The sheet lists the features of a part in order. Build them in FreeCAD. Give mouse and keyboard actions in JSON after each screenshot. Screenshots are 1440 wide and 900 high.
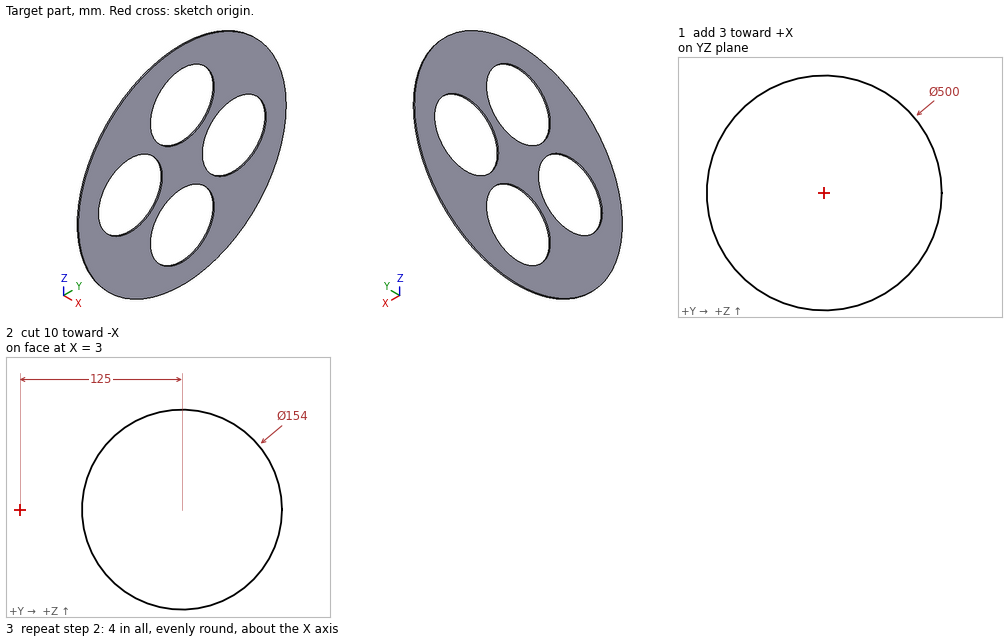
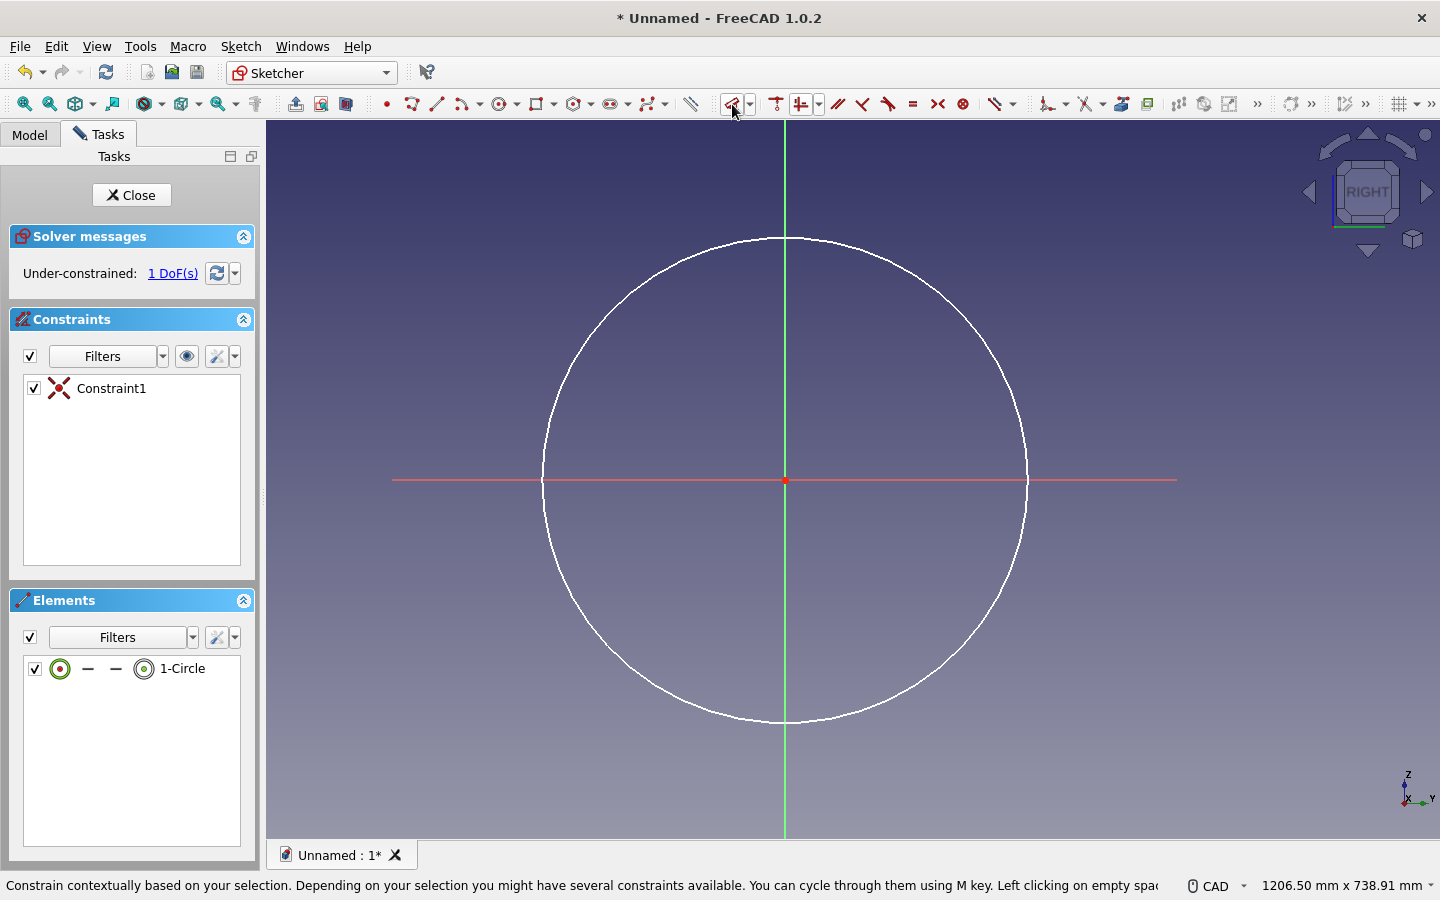
{"action": "left_click", "coordinate": [956, 308]}
{"action": "left_click", "coordinate": [979, 285]}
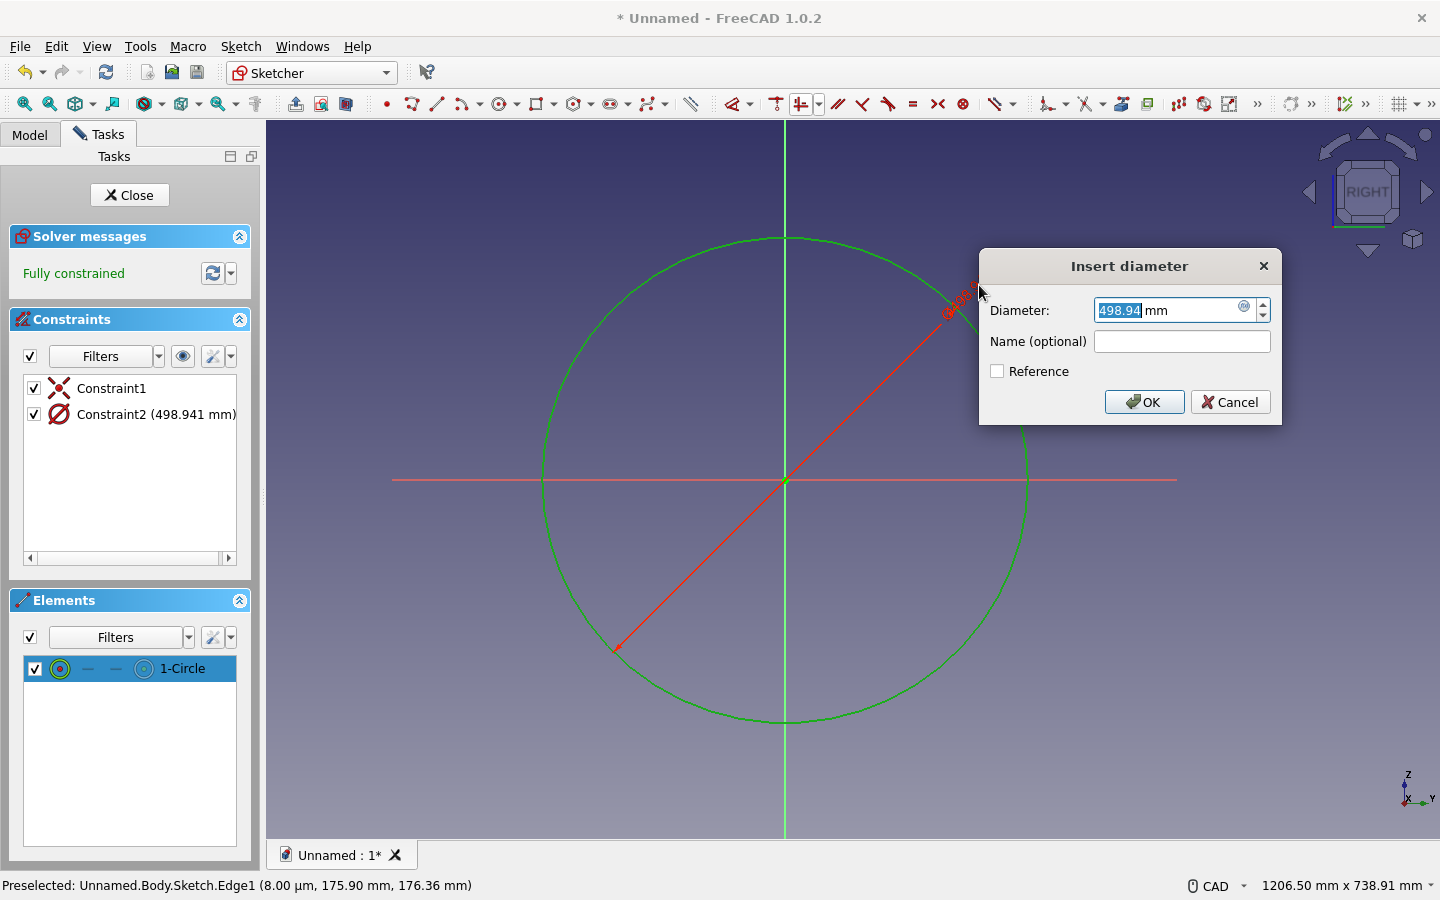
{"action": "type", "text": "500"}
{"action": "key", "text": "Return"}
{"action": "key", "text": "Escape"}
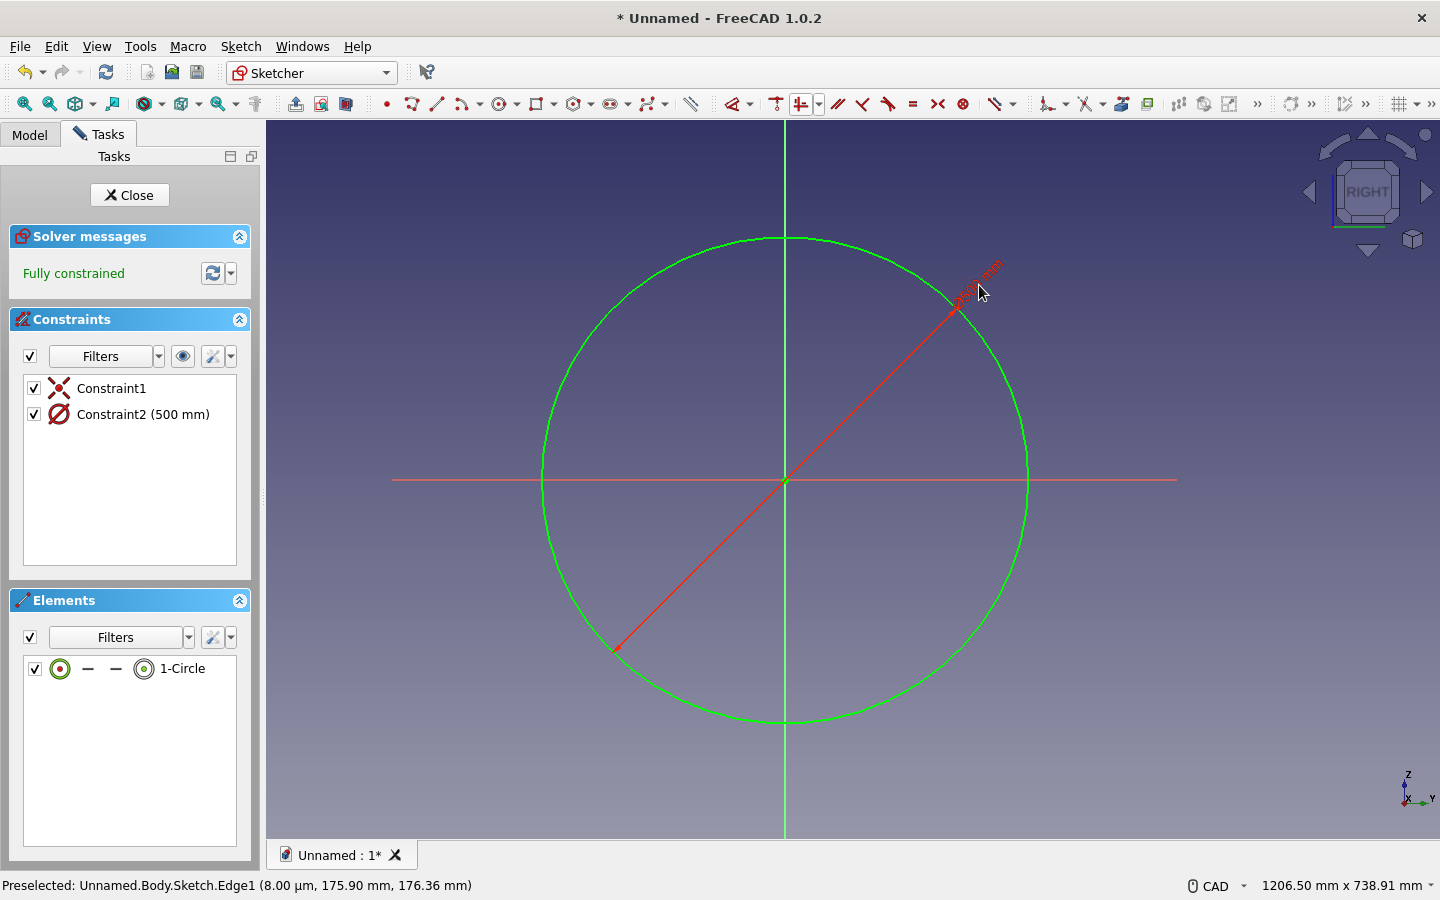
{"action": "left_click", "coordinate": [130, 195]}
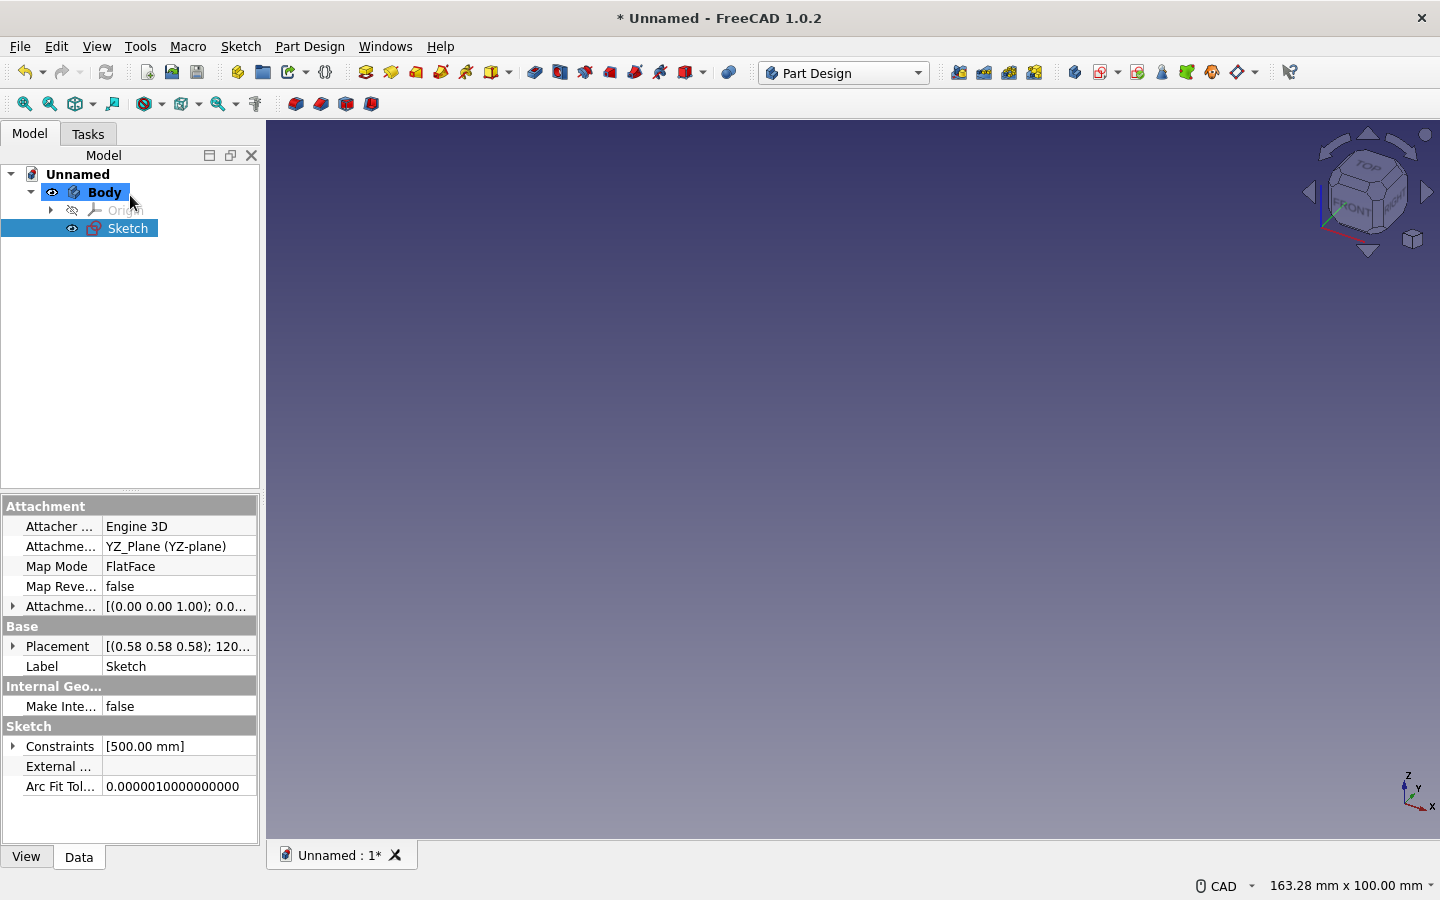
{"action": "left_click", "coordinate": [366, 72]}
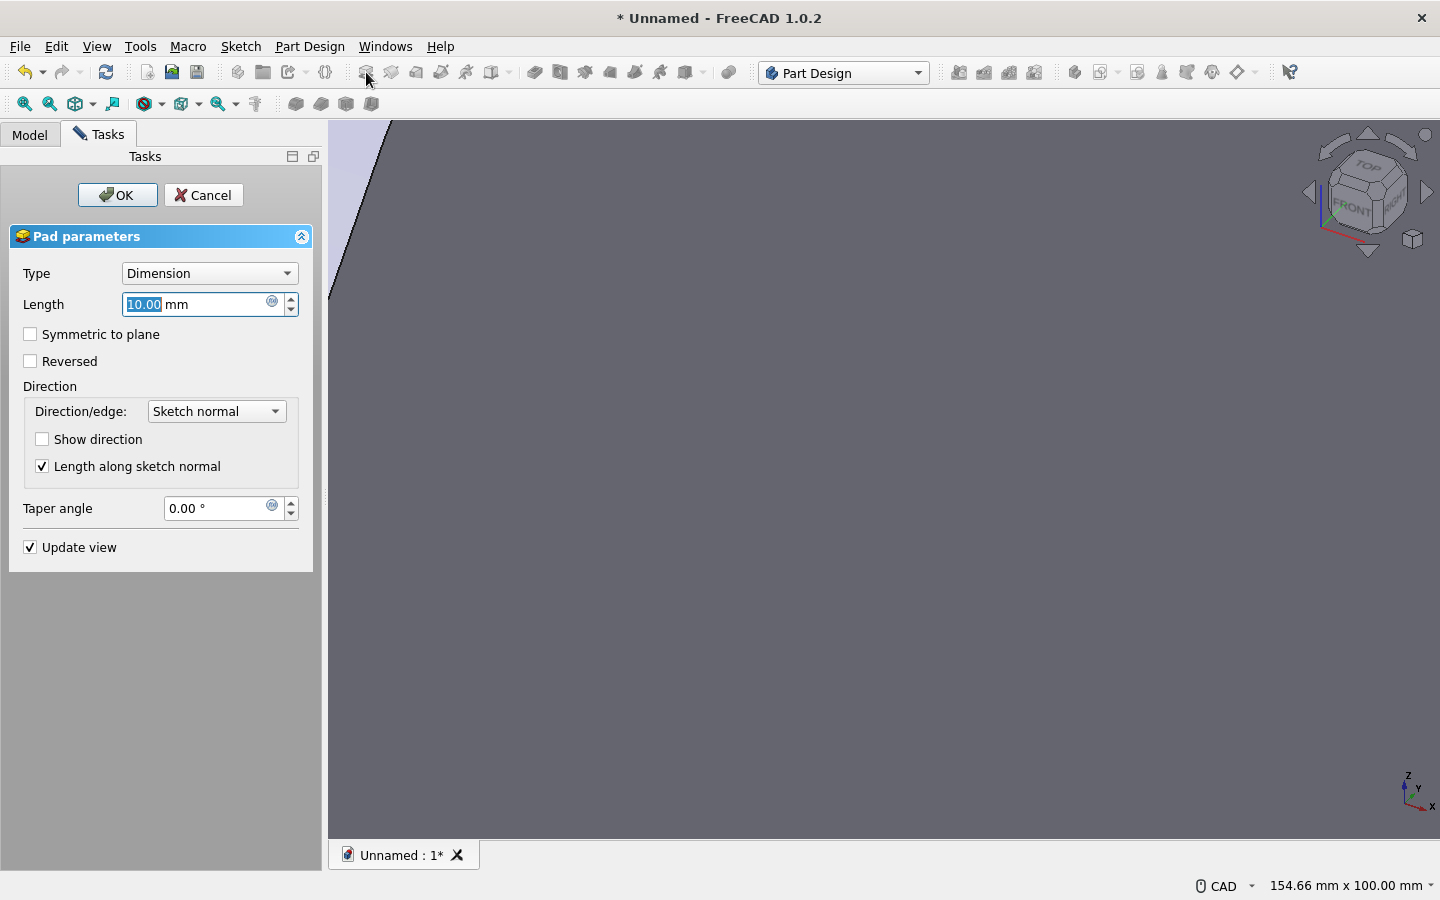
{"action": "type", "text": "3"}
{"action": "key", "text": "Tab"}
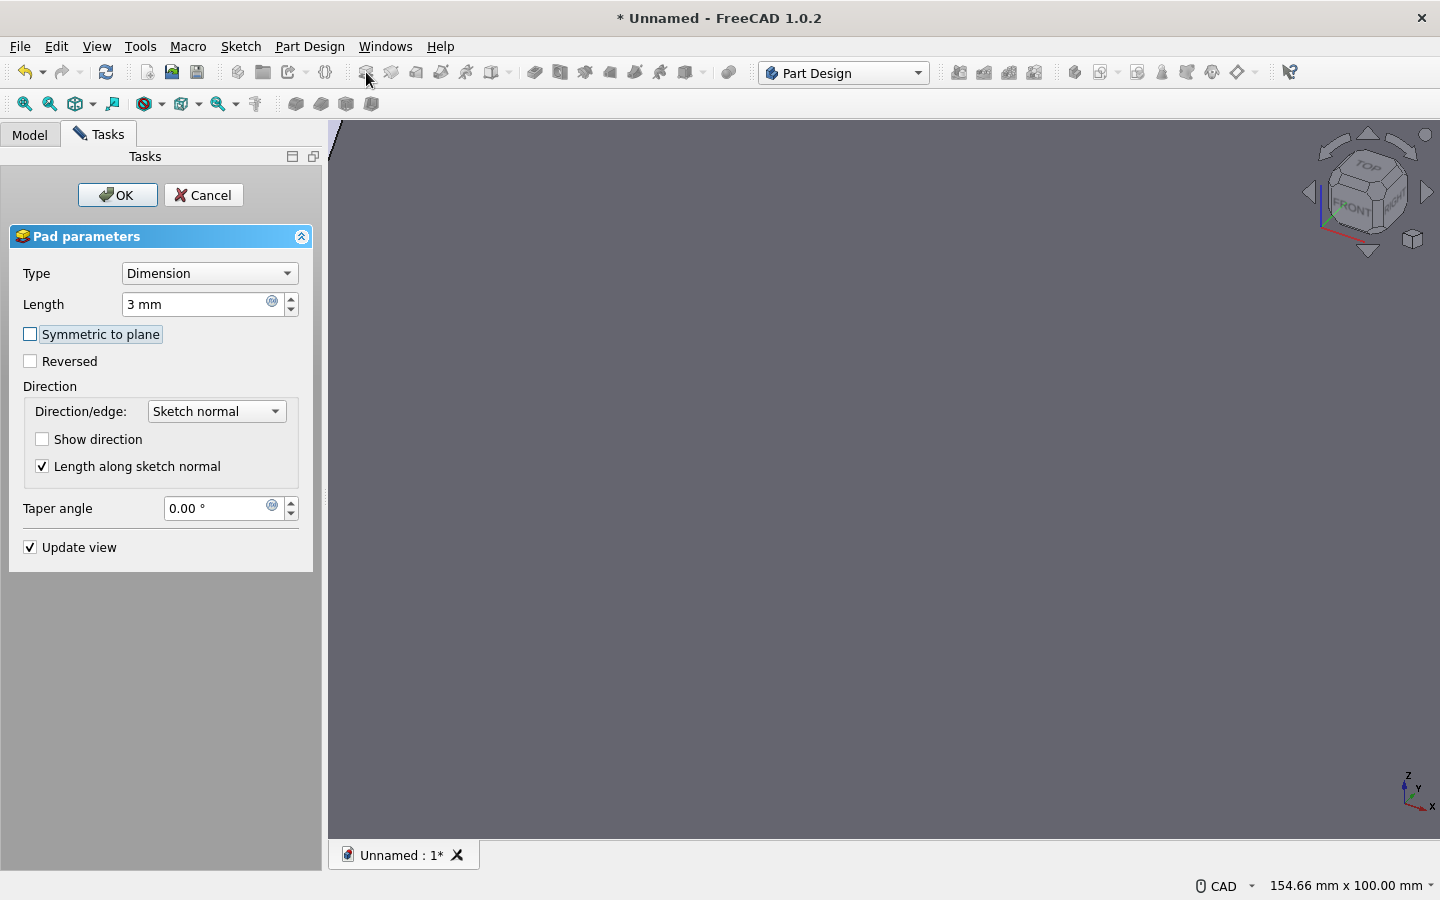
{"action": "left_click", "coordinate": [118, 195]}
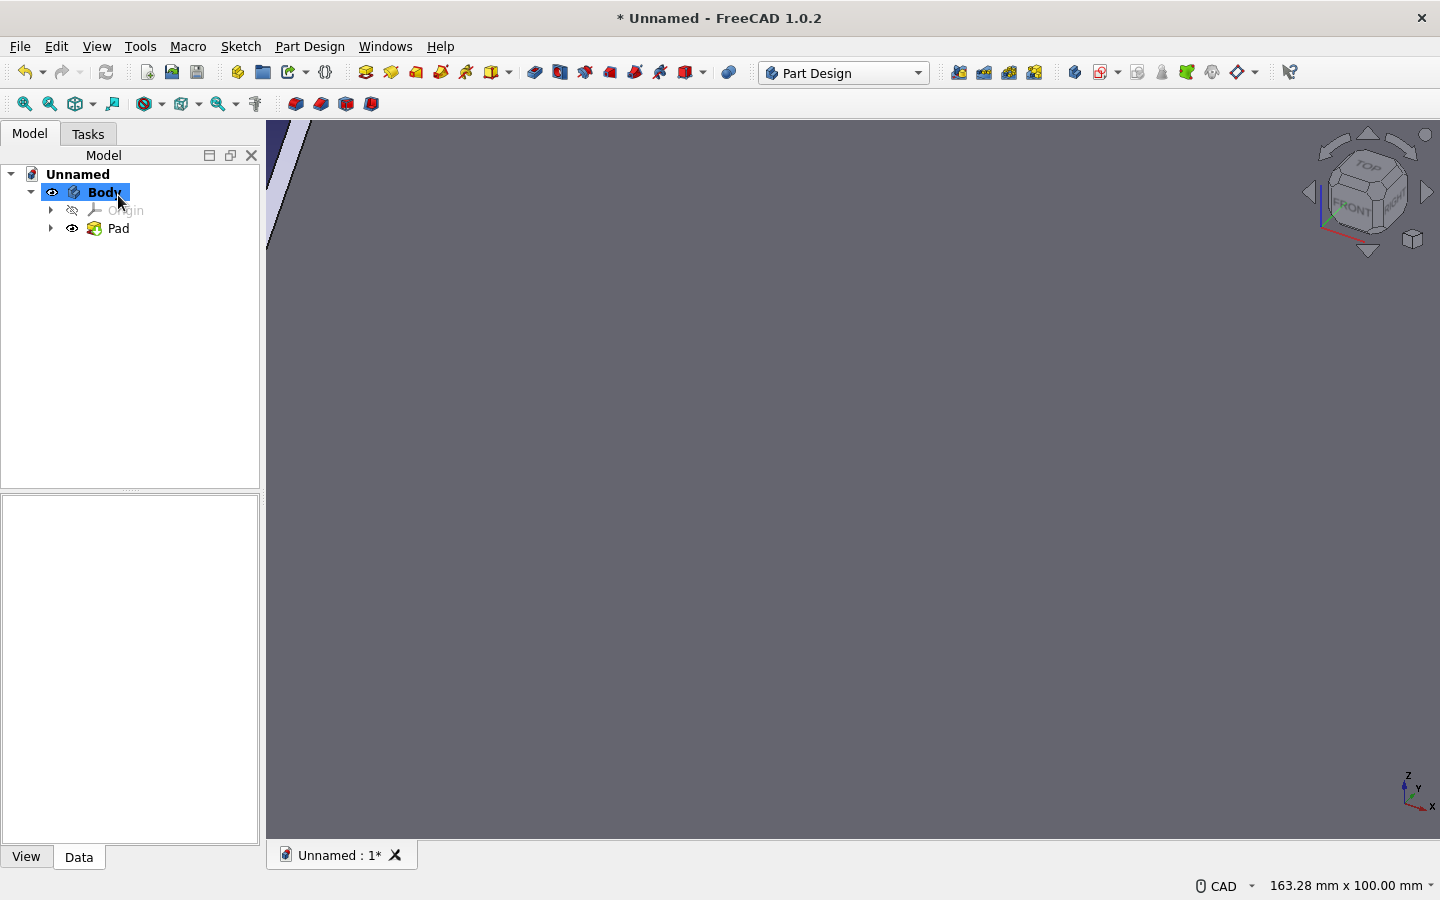
{"action": "left_click", "coordinate": [25, 104]}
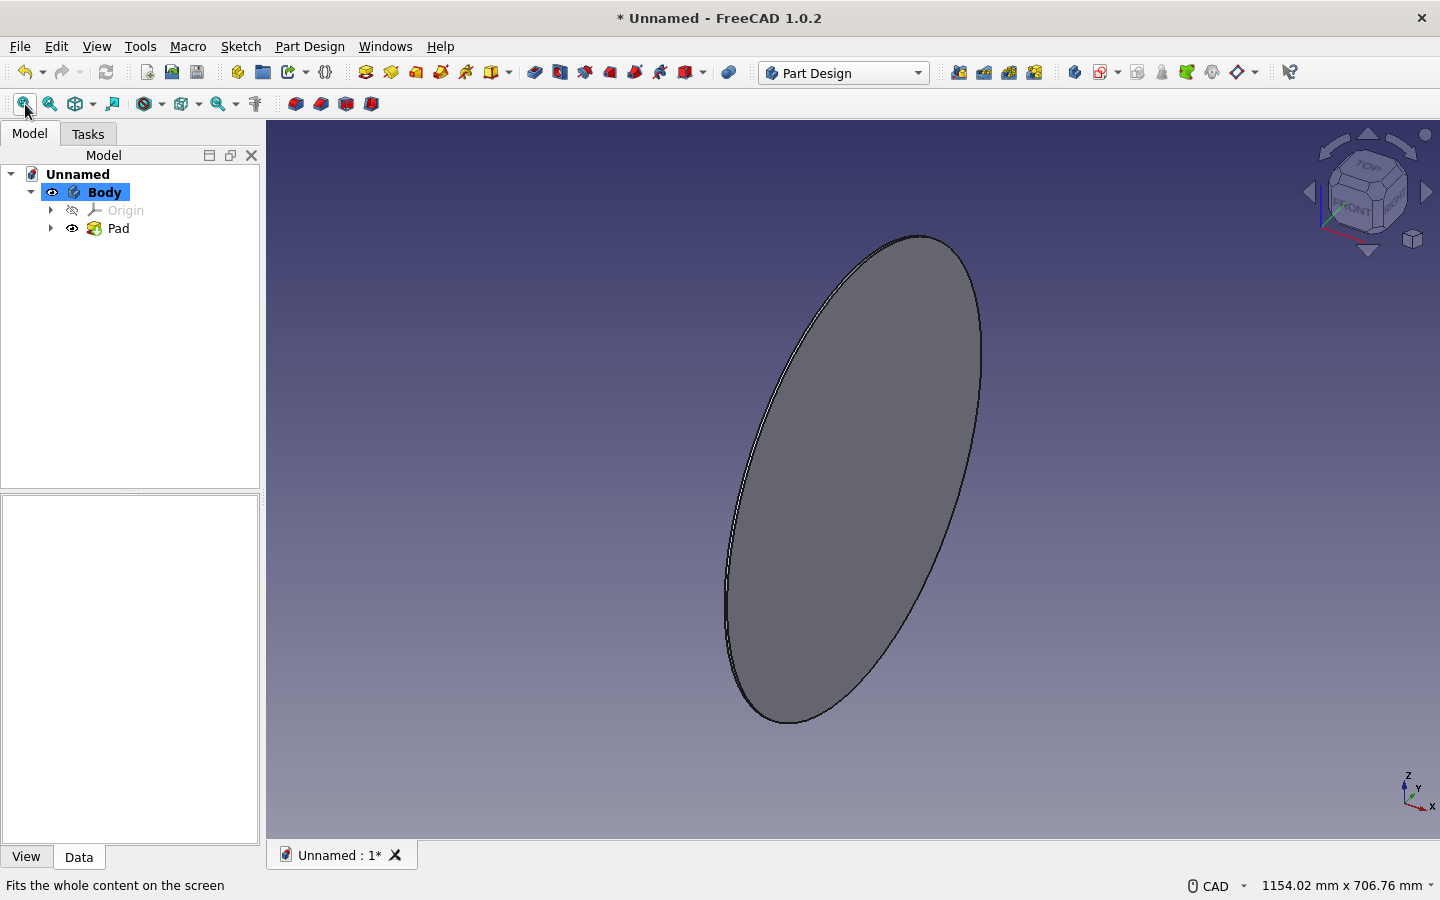
{"action": "left_click", "coordinate": [854, 479]}